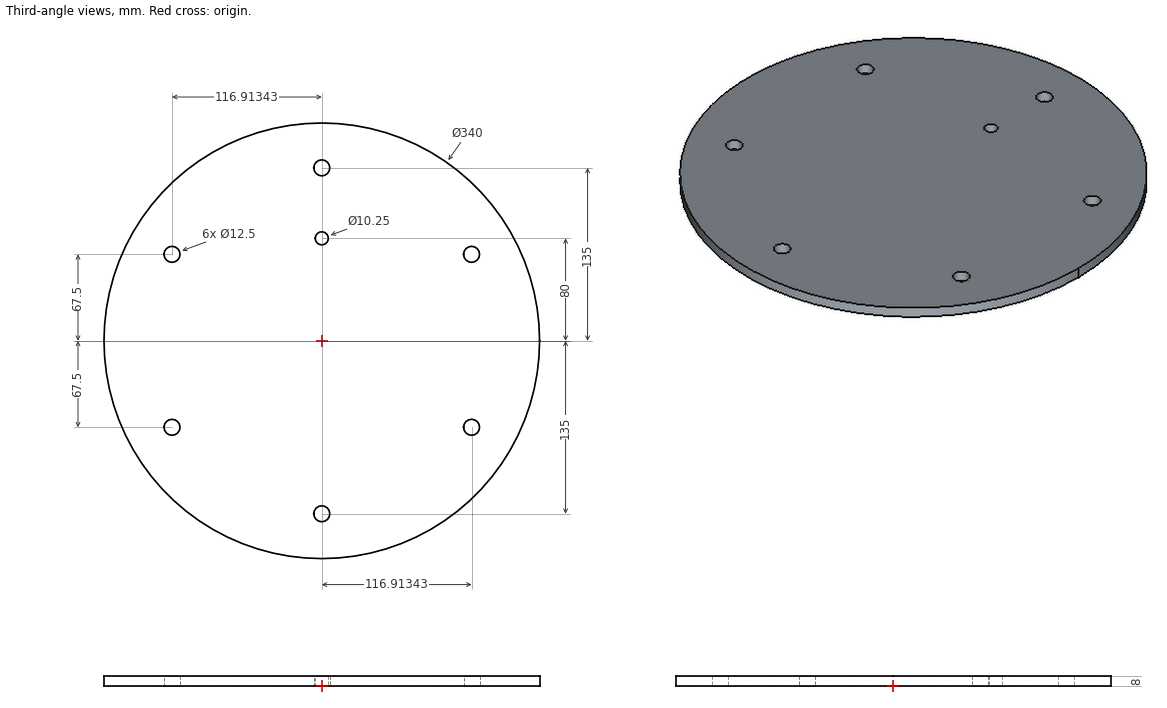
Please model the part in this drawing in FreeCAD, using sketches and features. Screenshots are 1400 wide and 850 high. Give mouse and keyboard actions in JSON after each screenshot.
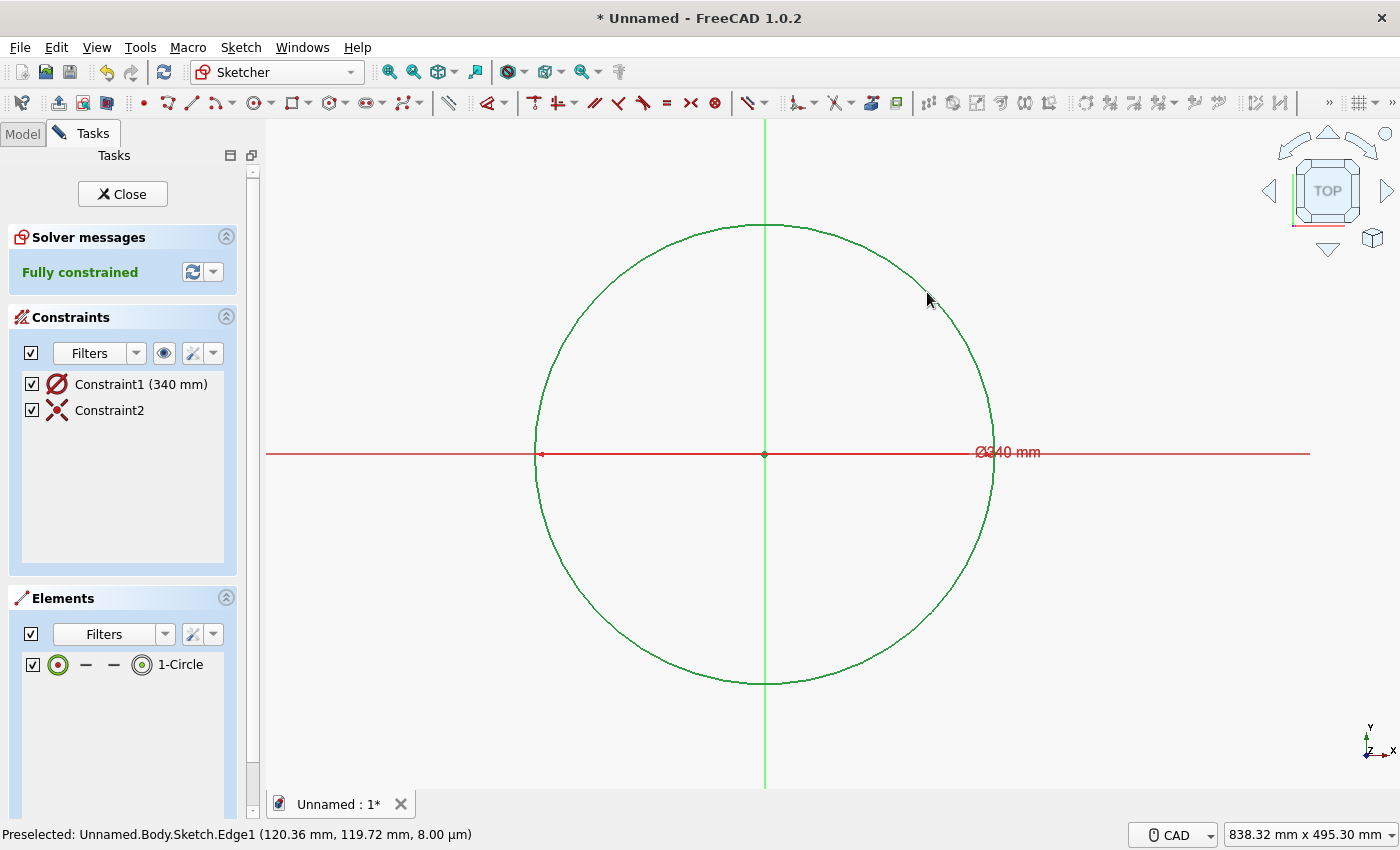
{"action": "left_click", "coordinate": [123, 194]}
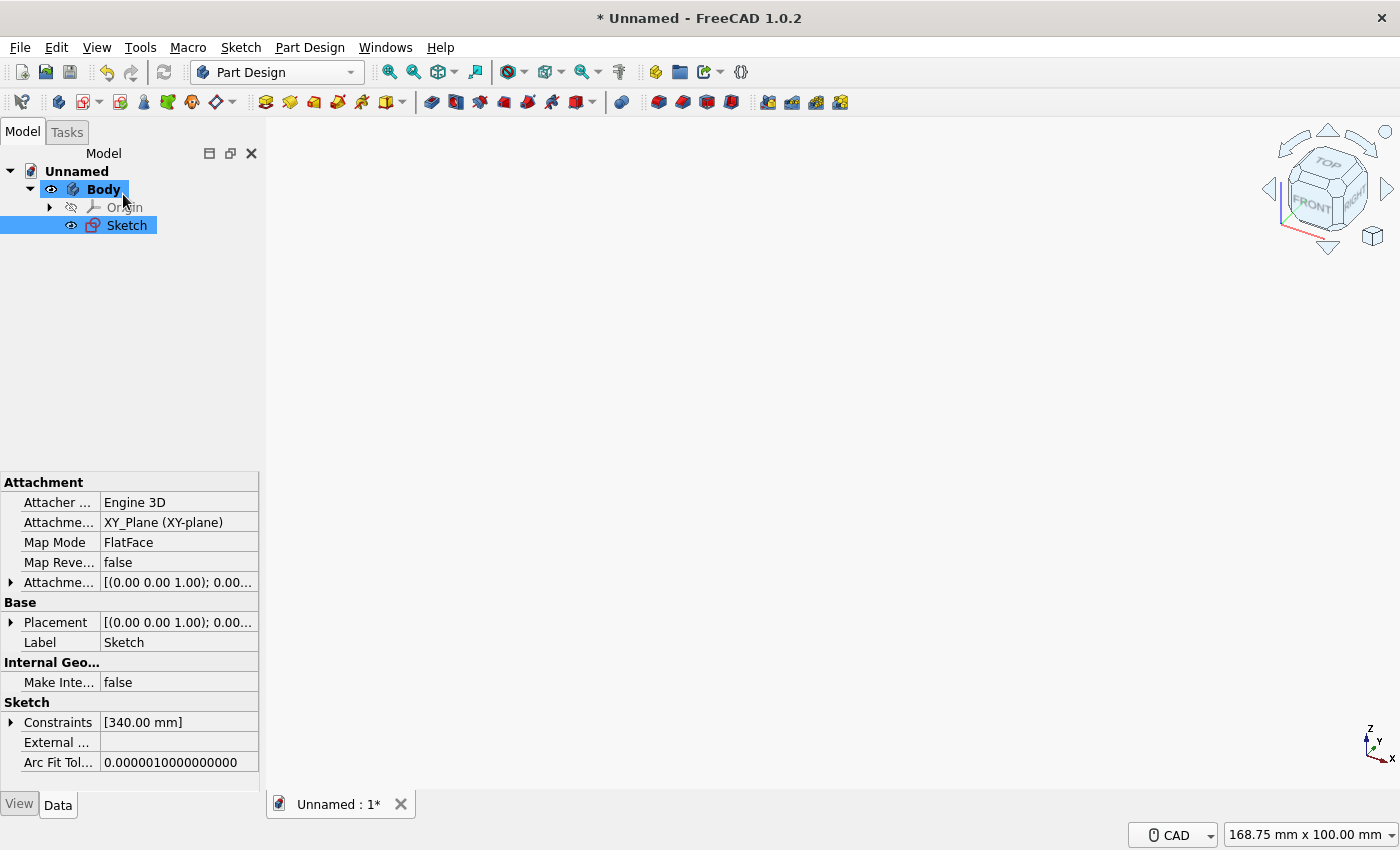
{"action": "left_click", "coordinate": [266, 102]}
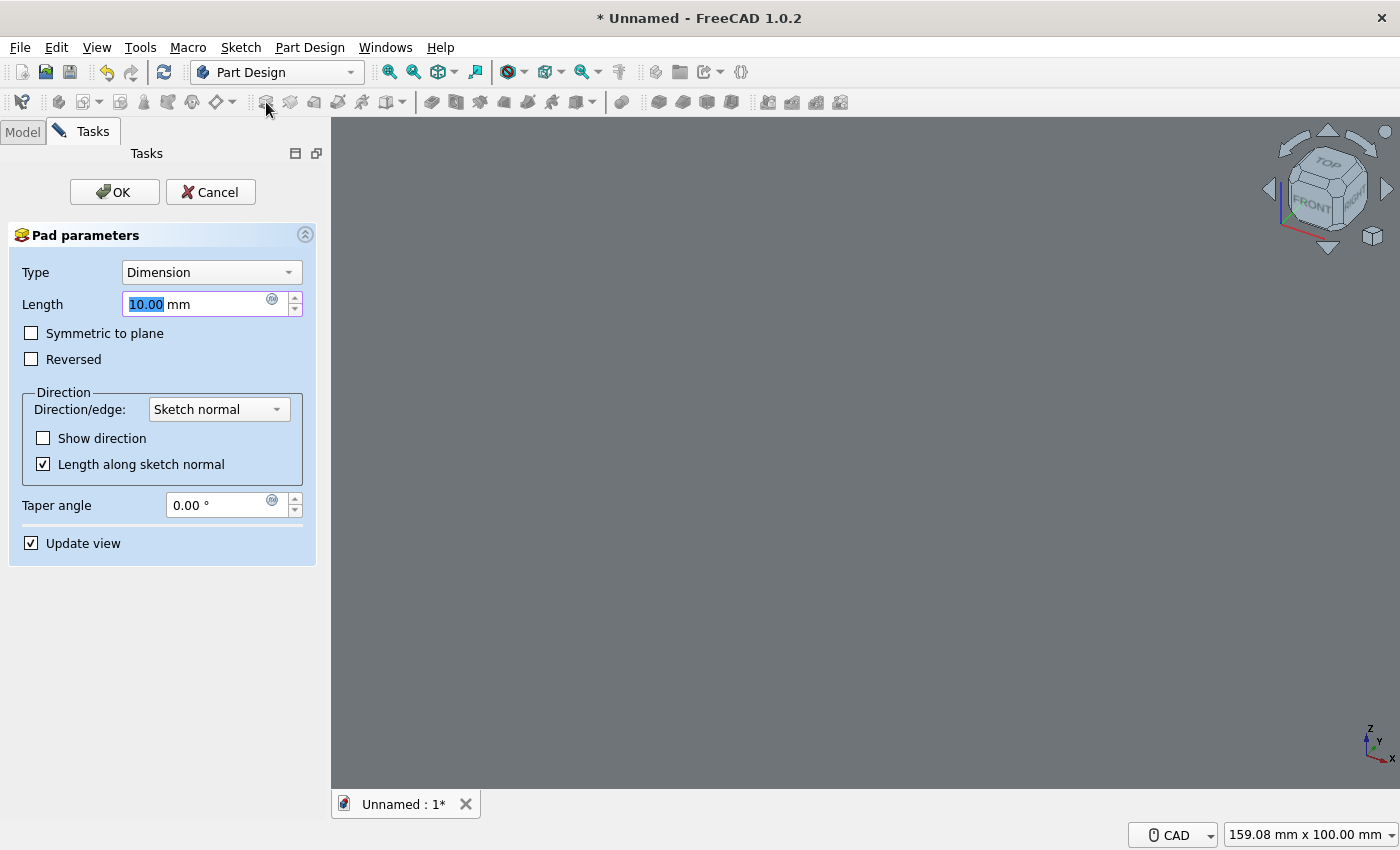
{"action": "type", "text": "8"}
{"action": "key", "text": "Tab"}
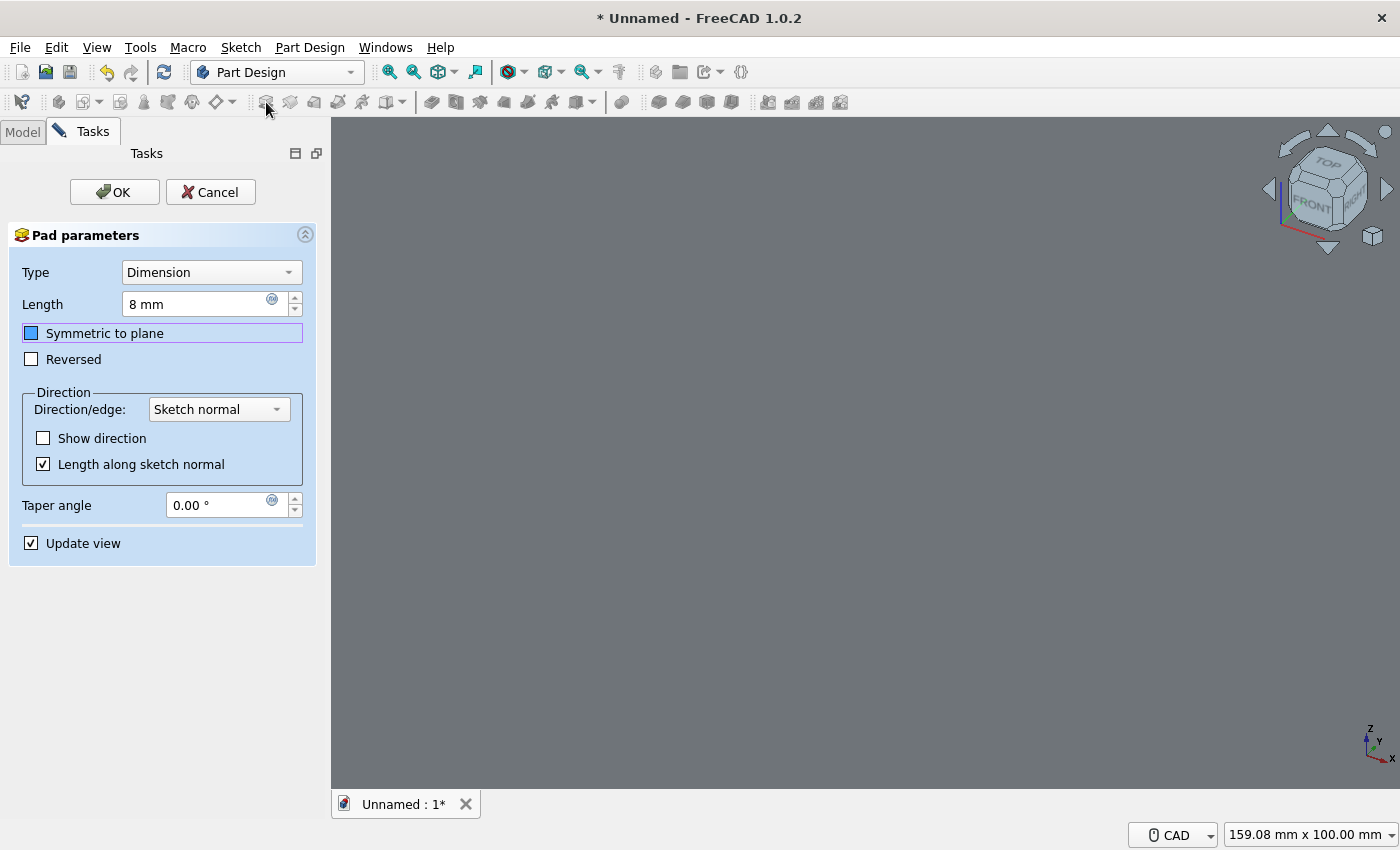
{"action": "left_click", "coordinate": [115, 192]}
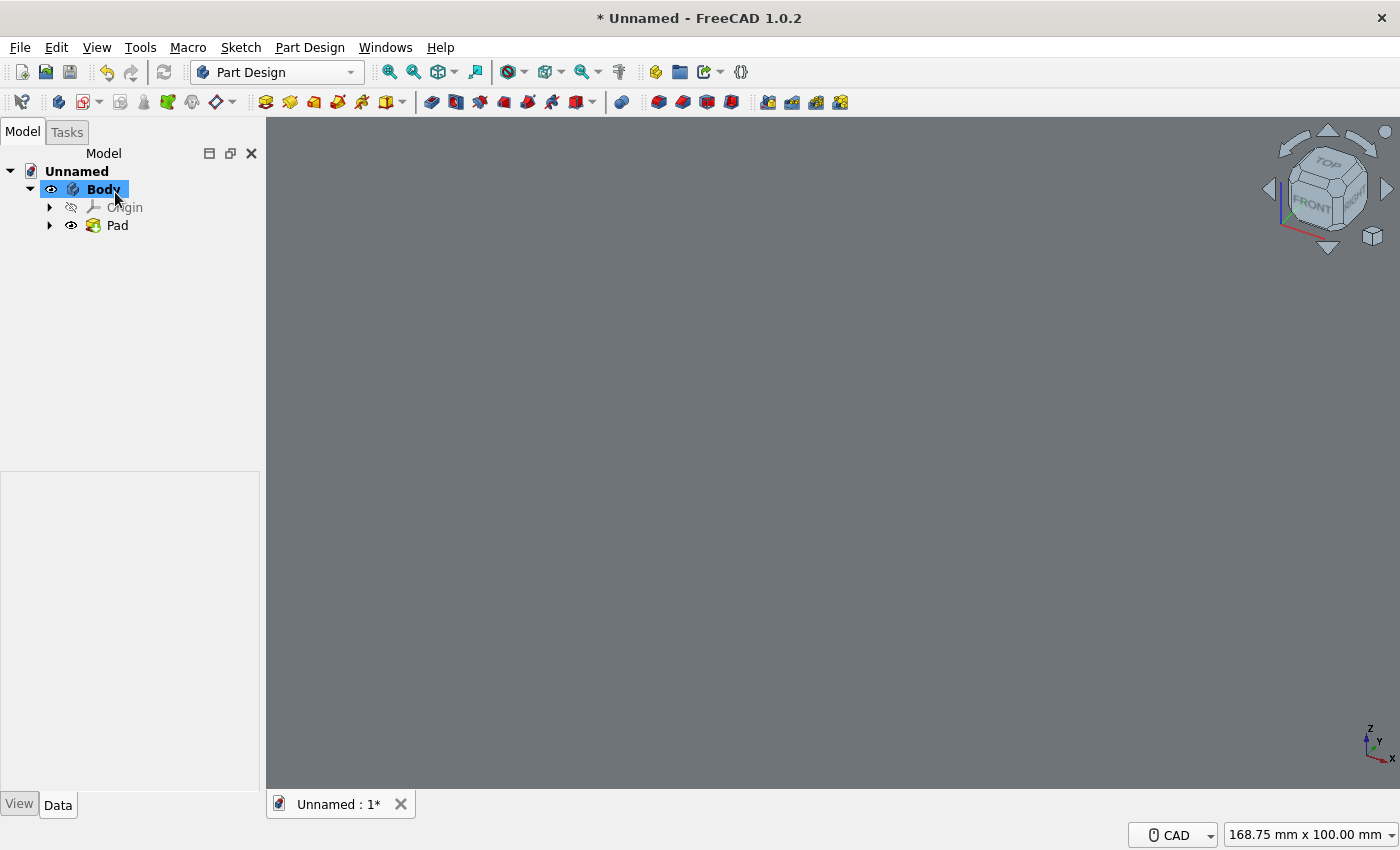
{"action": "left_click", "coordinate": [390, 72]}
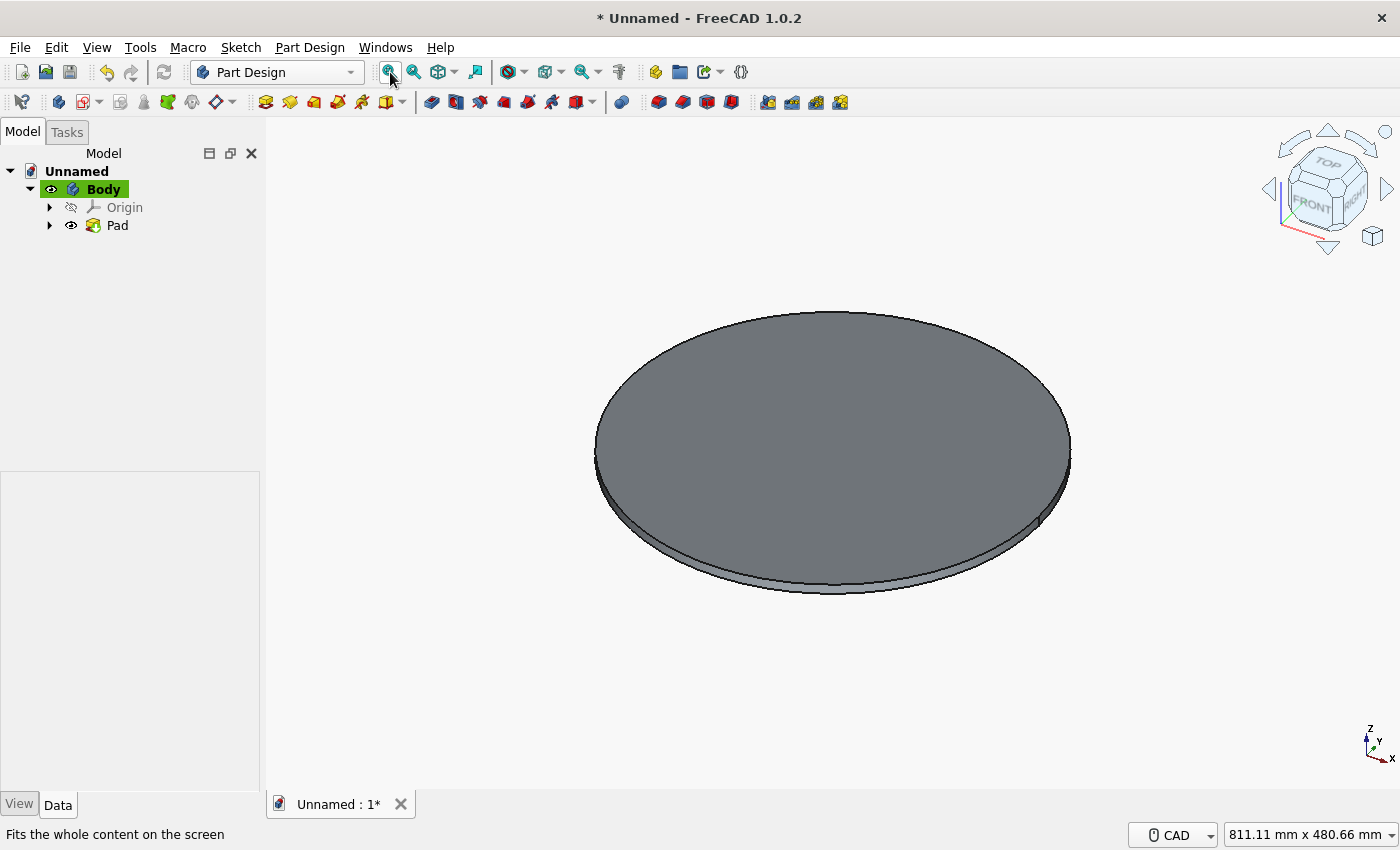
{"action": "key", "text": "5"}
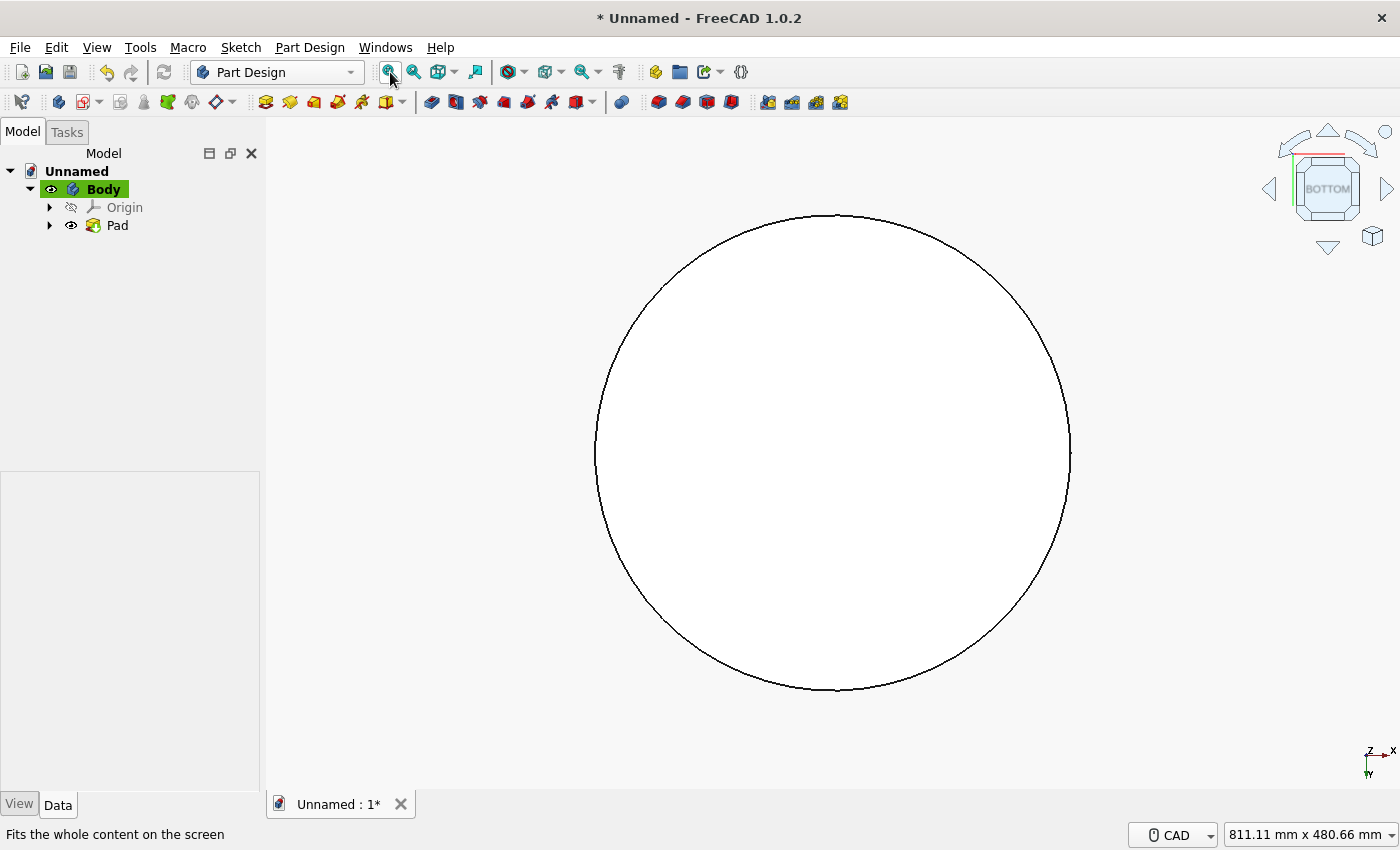
{"action": "left_click", "coordinate": [833, 452]}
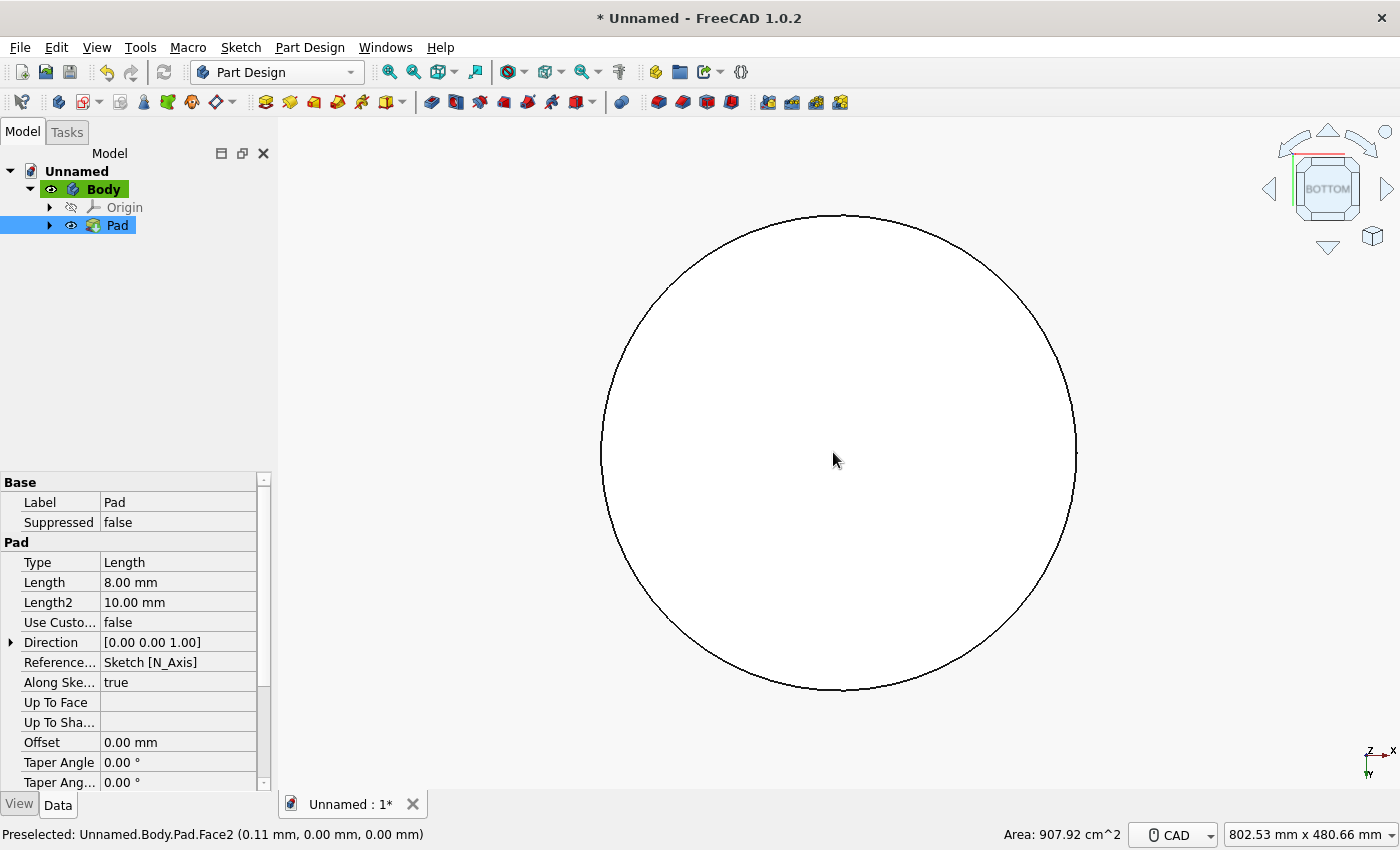
{"action": "left_click", "coordinate": [84, 102]}